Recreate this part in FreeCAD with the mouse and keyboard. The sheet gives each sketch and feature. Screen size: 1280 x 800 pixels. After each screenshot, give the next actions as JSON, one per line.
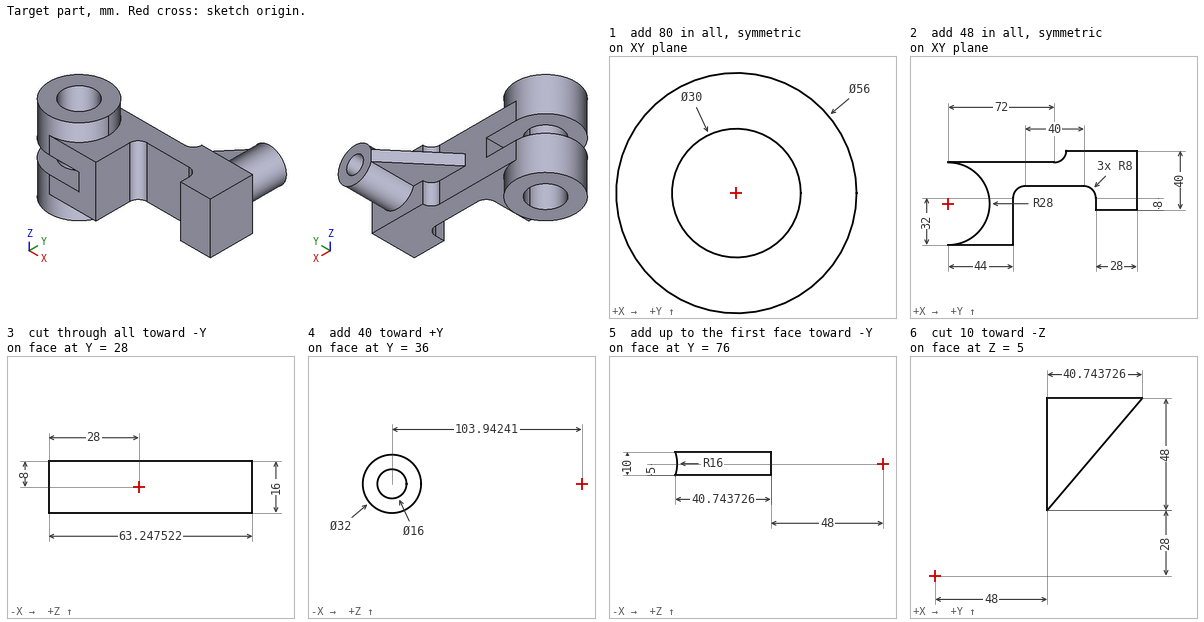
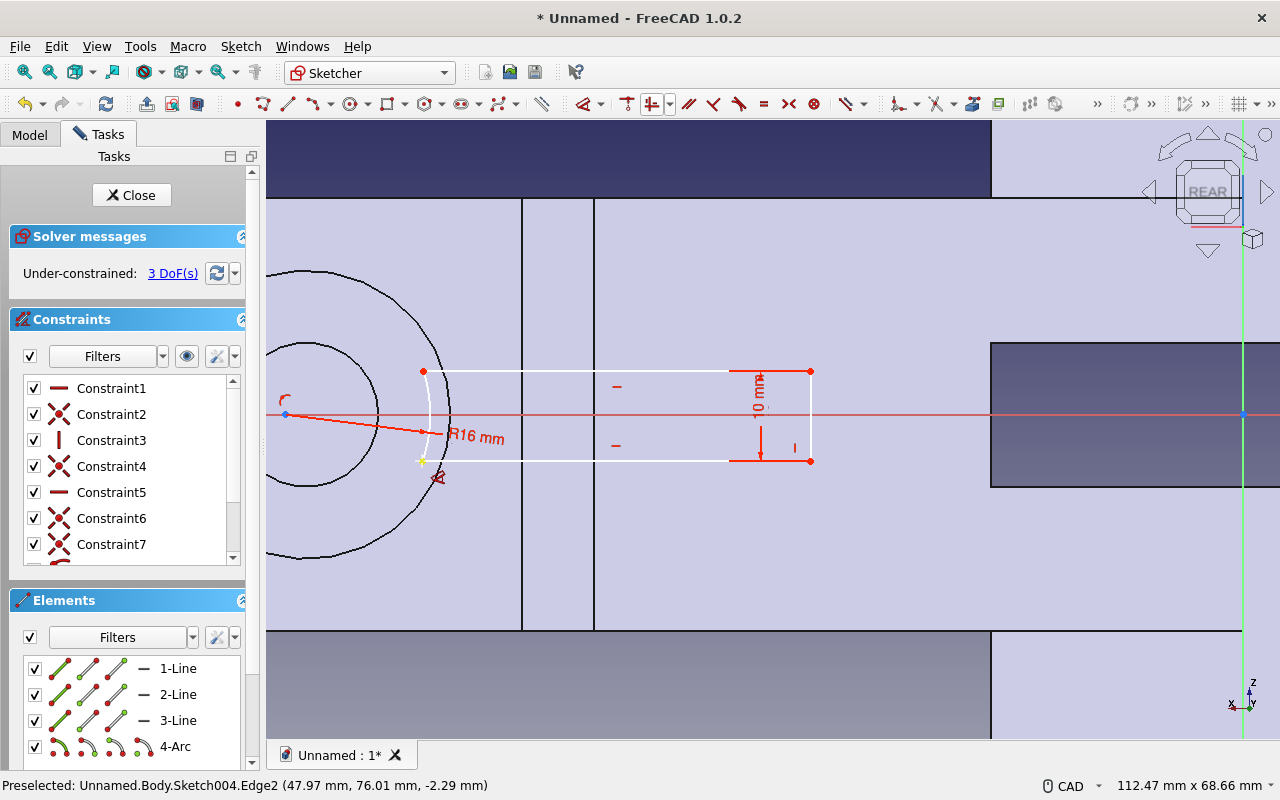
{"action": "left_click", "coordinate": [422, 461]}
{"action": "left_click", "coordinate": [388, 438]}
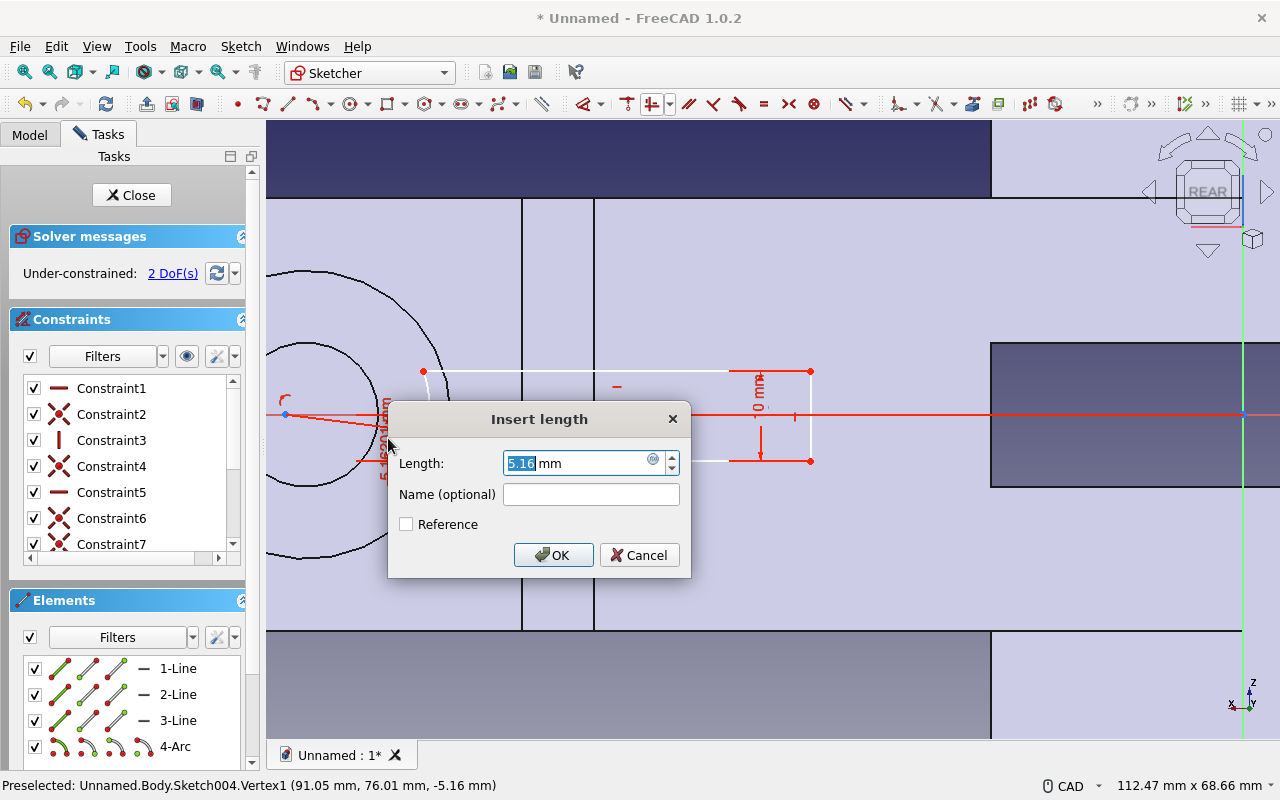
{"action": "type", "text": "5"}
{"action": "key", "text": "Return"}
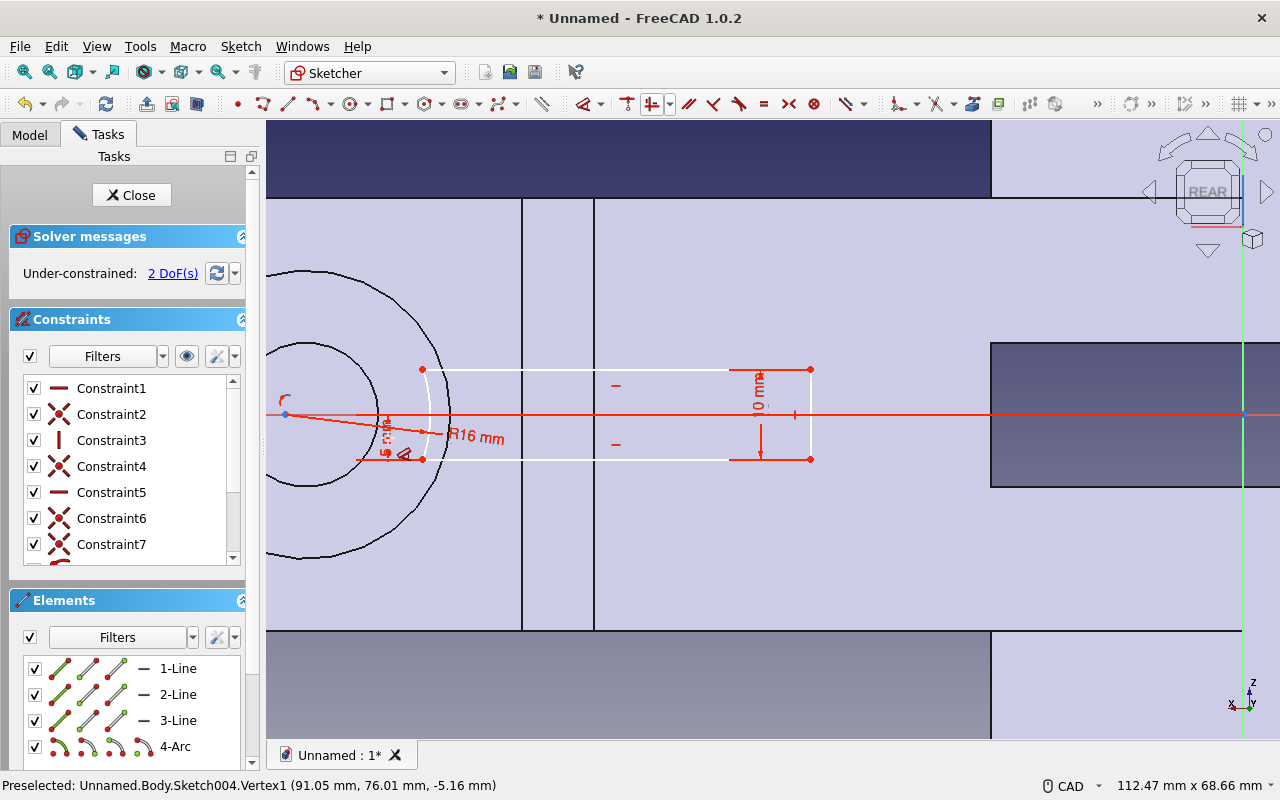
{"action": "left_click", "coordinate": [811, 460]}
{"action": "left_click", "coordinate": [963, 494]}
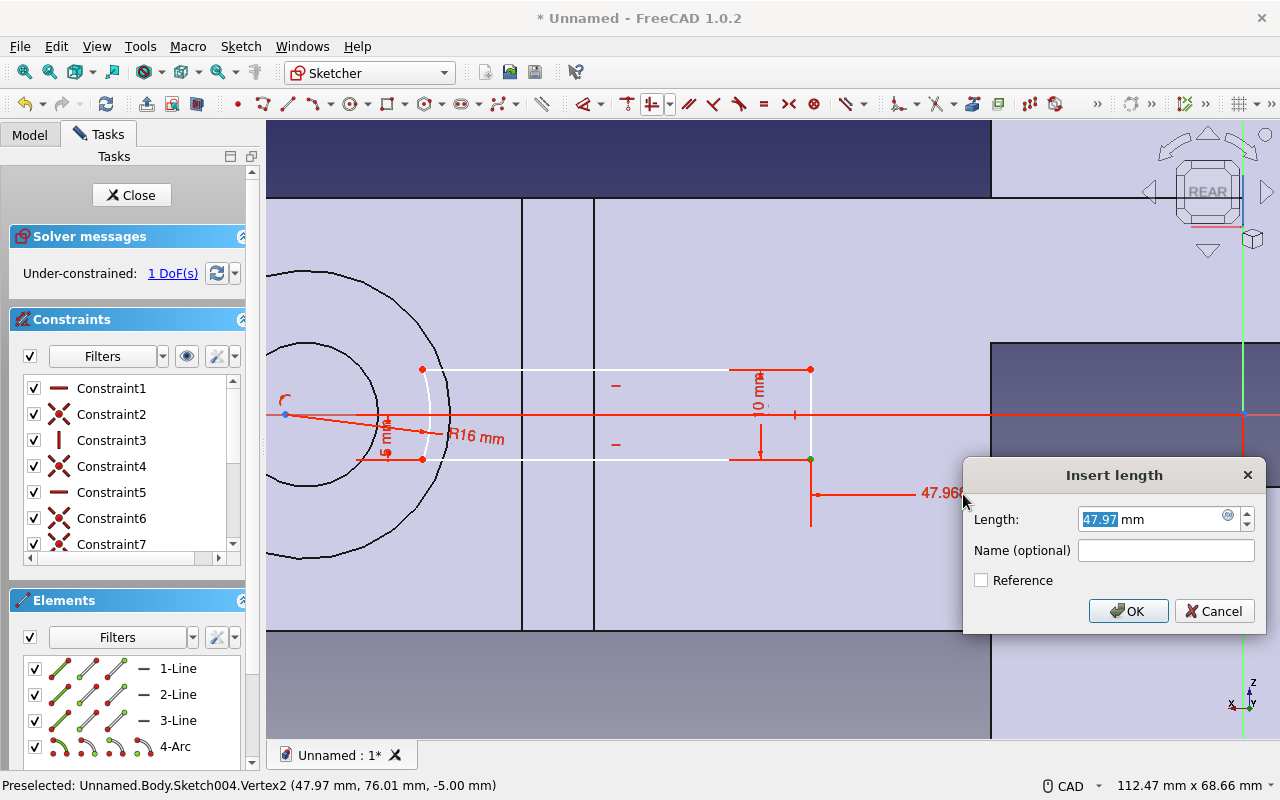
{"action": "type", "text": "48"}
{"action": "key", "text": "Return"}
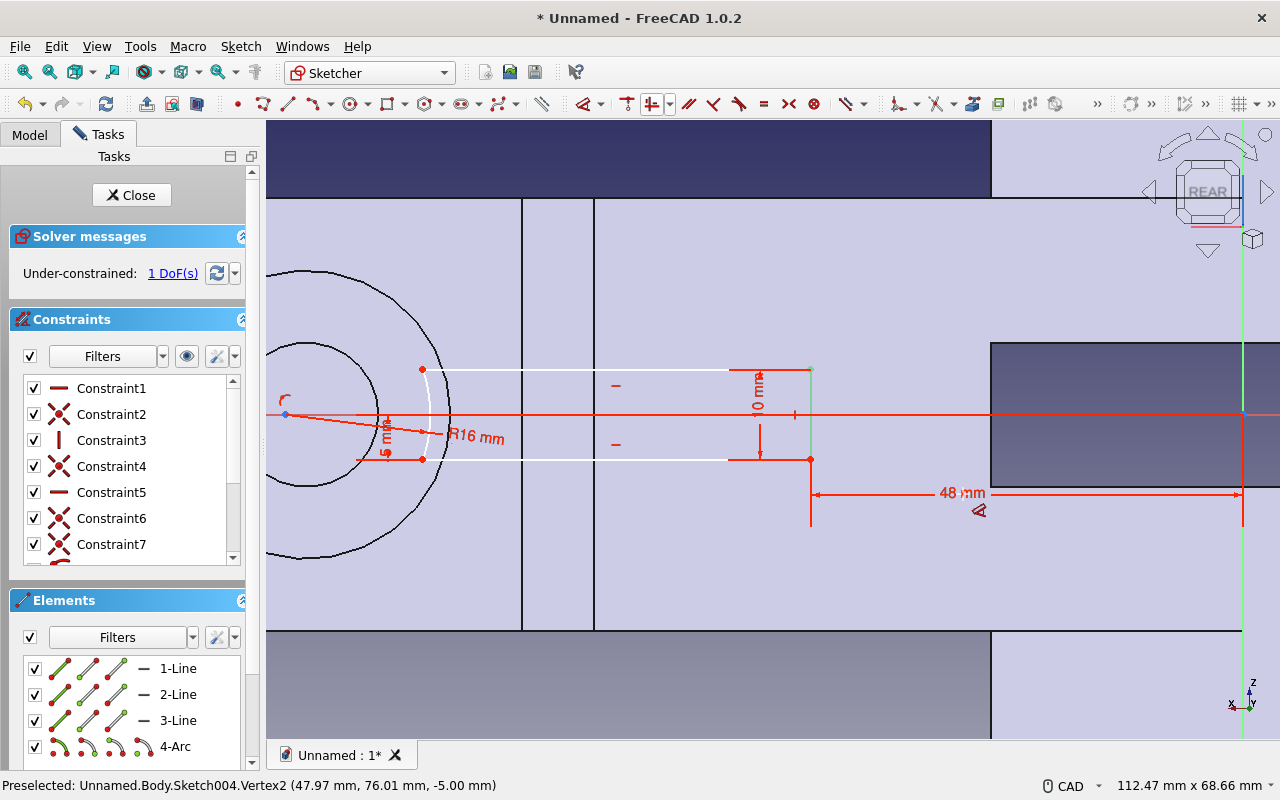
{"action": "left_click", "coordinate": [539, 460]}
{"action": "left_click", "coordinate": [617, 494]}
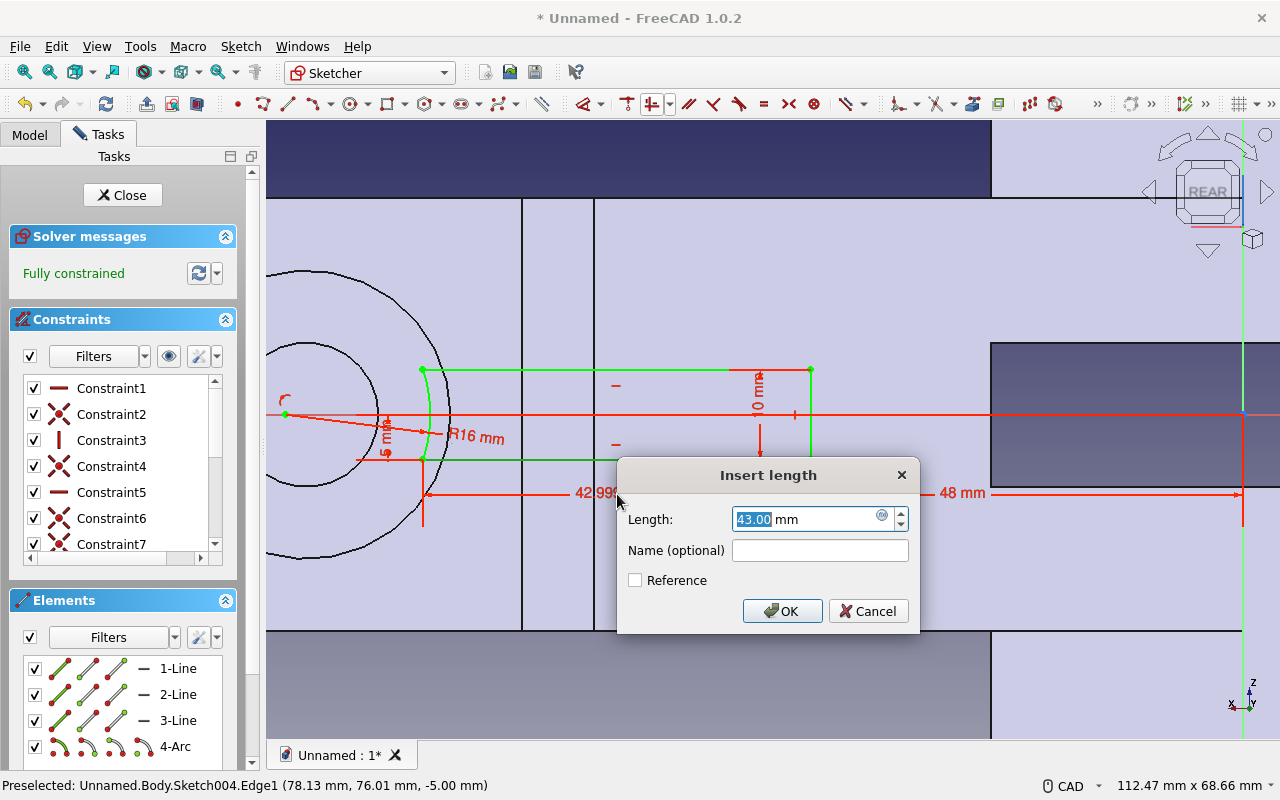
{"action": "type", "text": "40.743726"}
{"action": "key", "text": "Return"}
{"action": "key", "text": "Escape"}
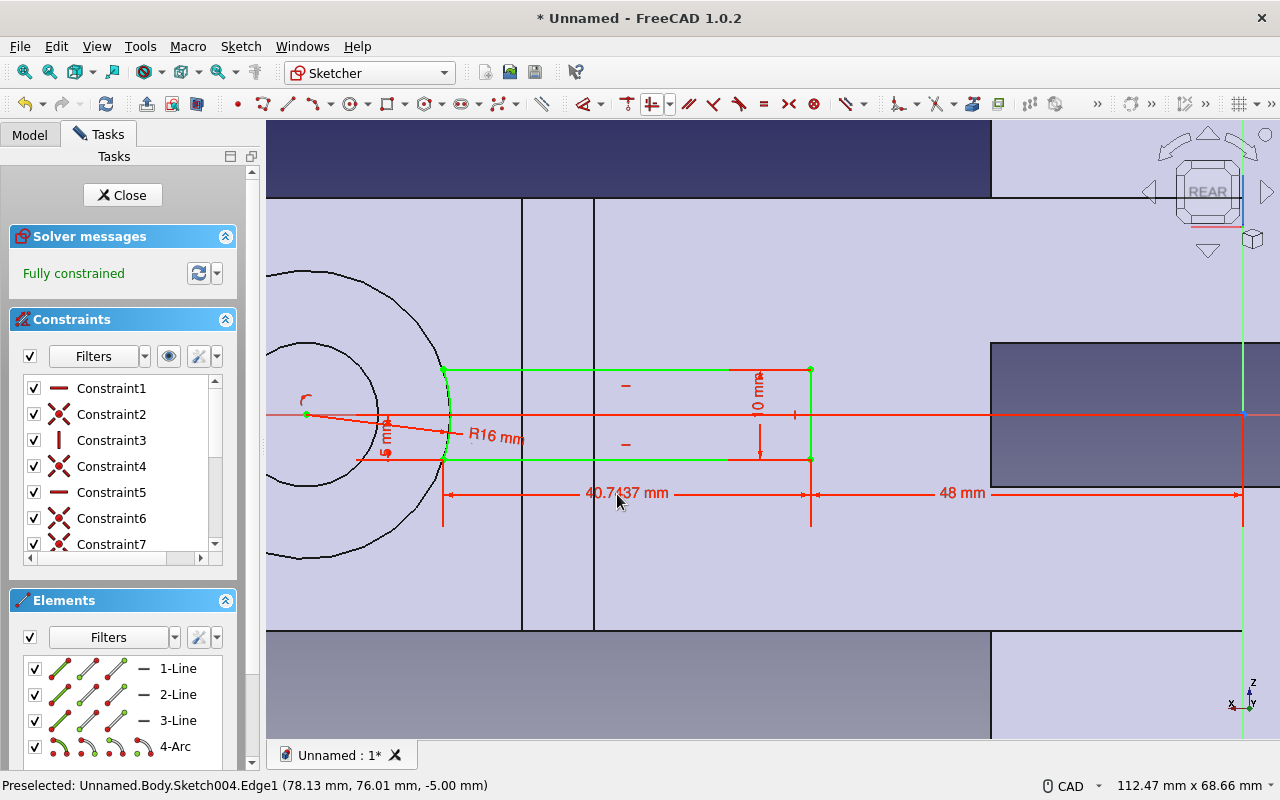
{"action": "left_click", "coordinate": [123, 195]}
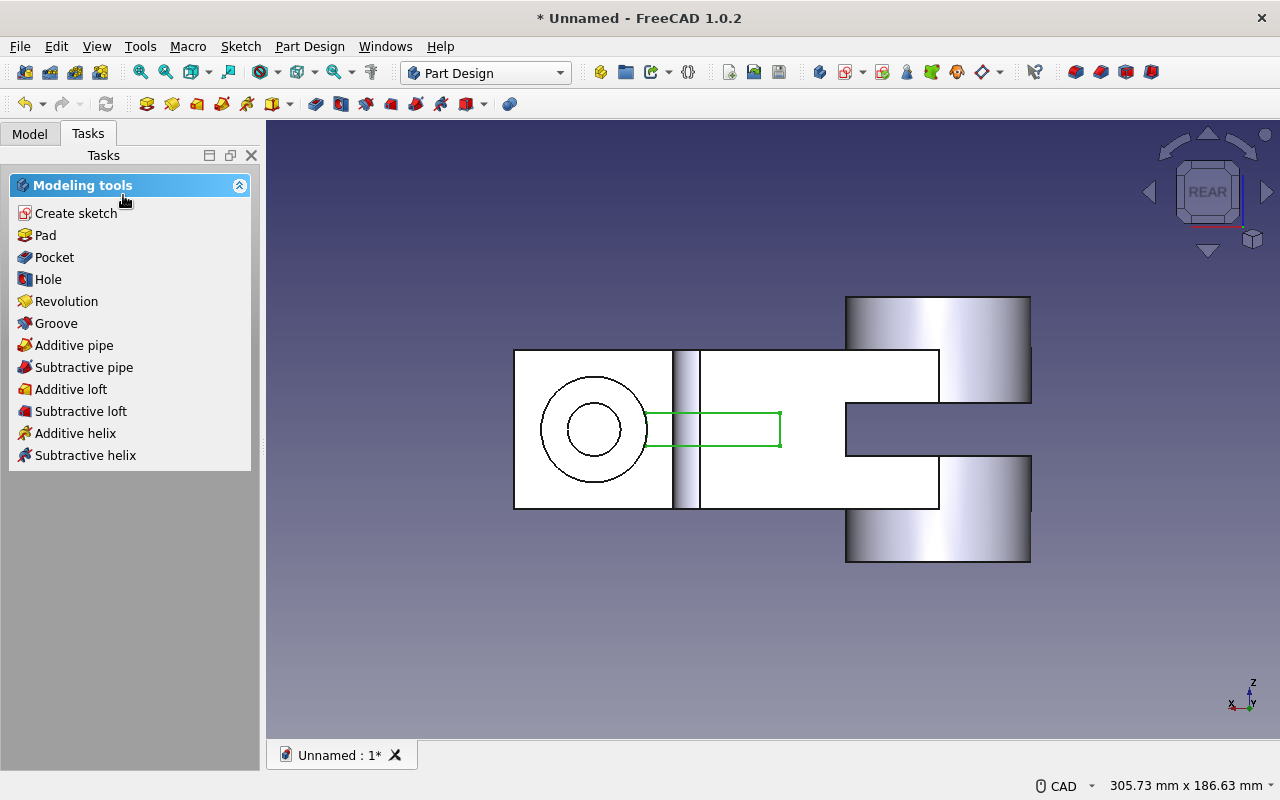
{"action": "left_click", "coordinate": [147, 104]}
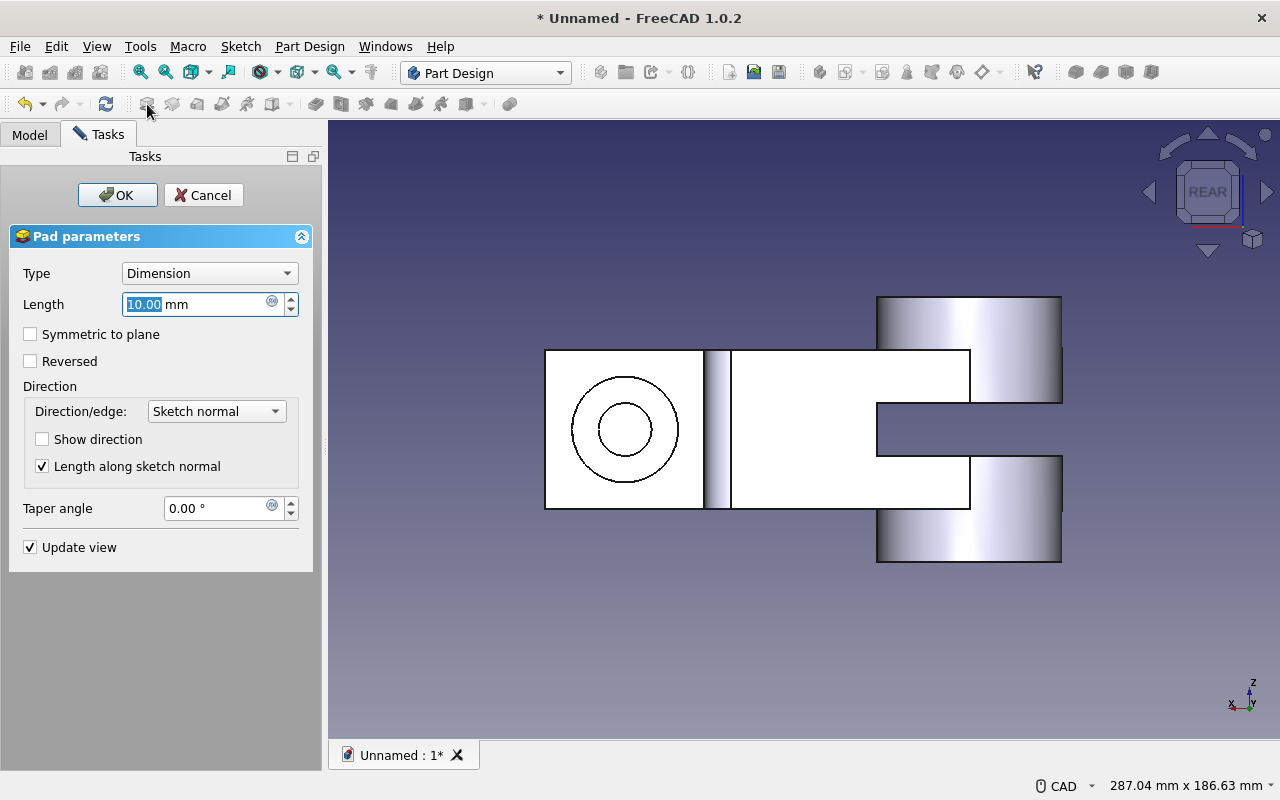
{"action": "left_click", "coordinate": [210, 274]}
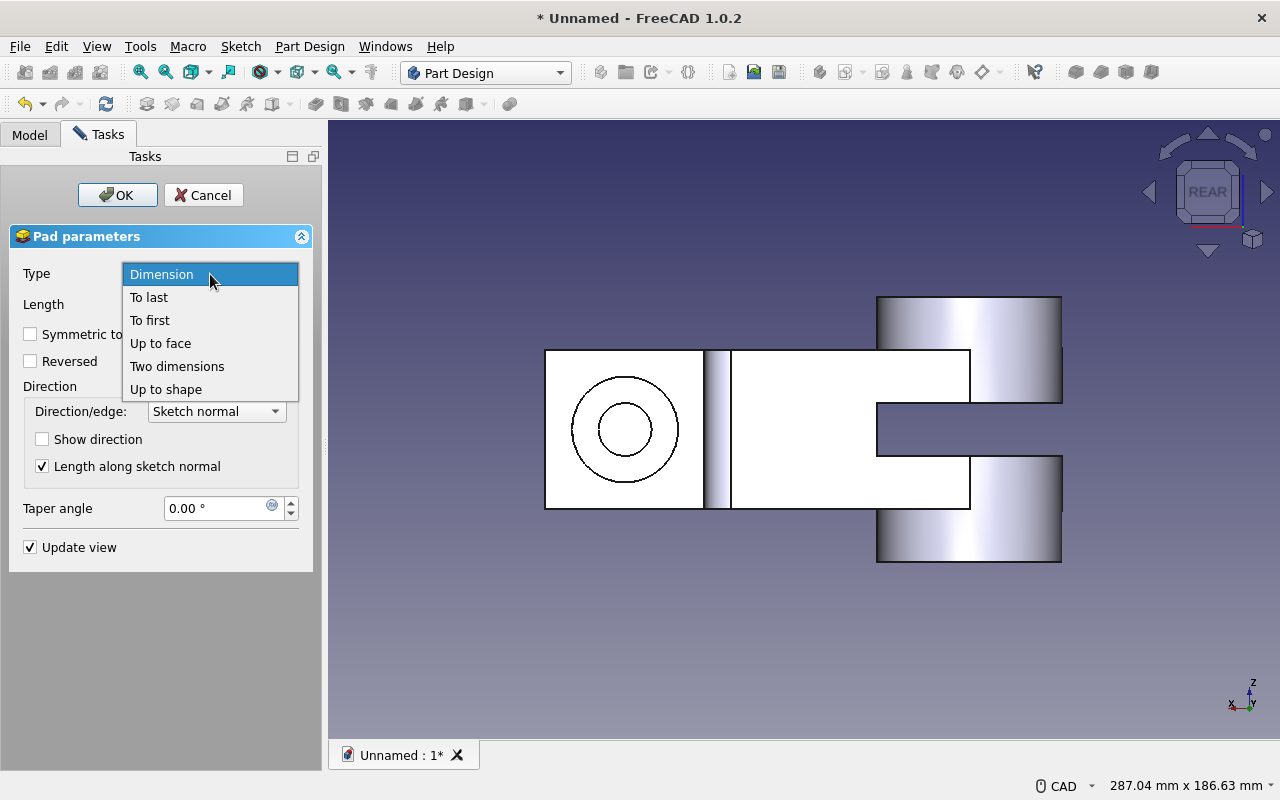
{"action": "left_click", "coordinate": [208, 320]}